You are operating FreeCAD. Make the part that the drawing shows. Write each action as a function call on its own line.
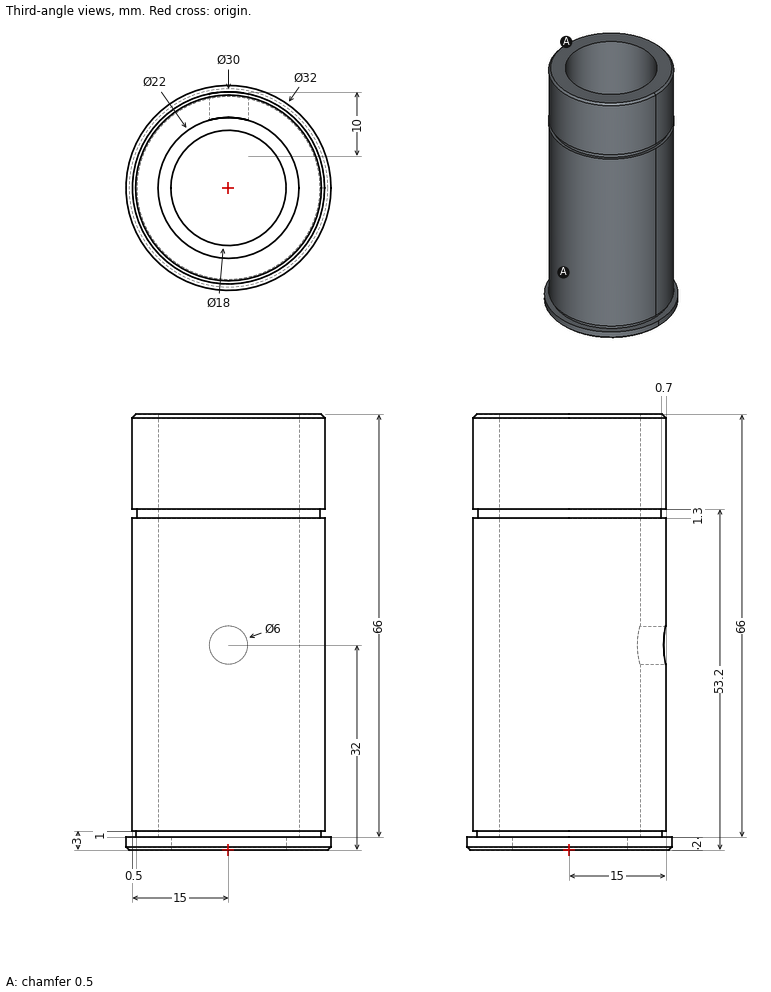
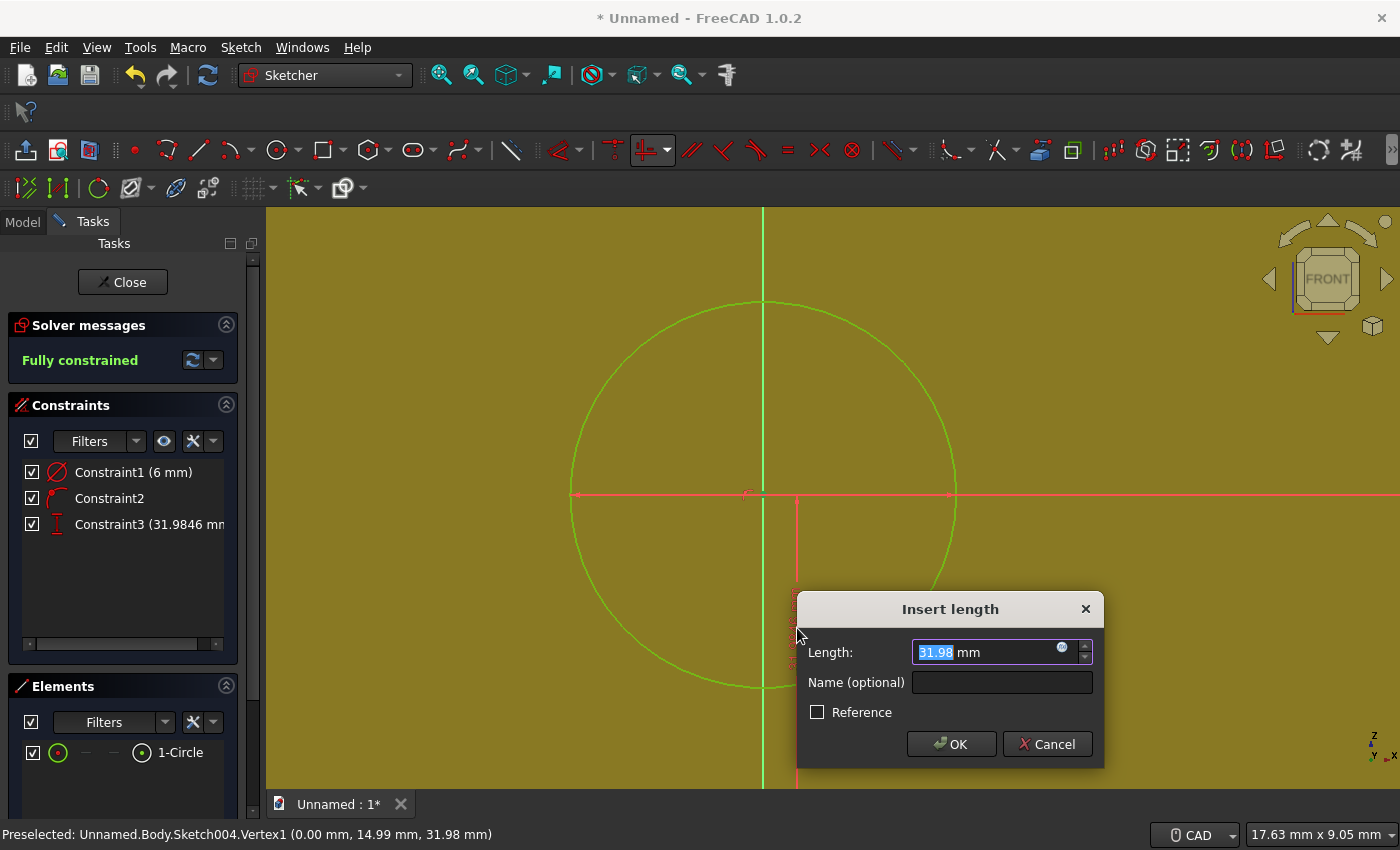
text(32)
key(Return)
key(Escape)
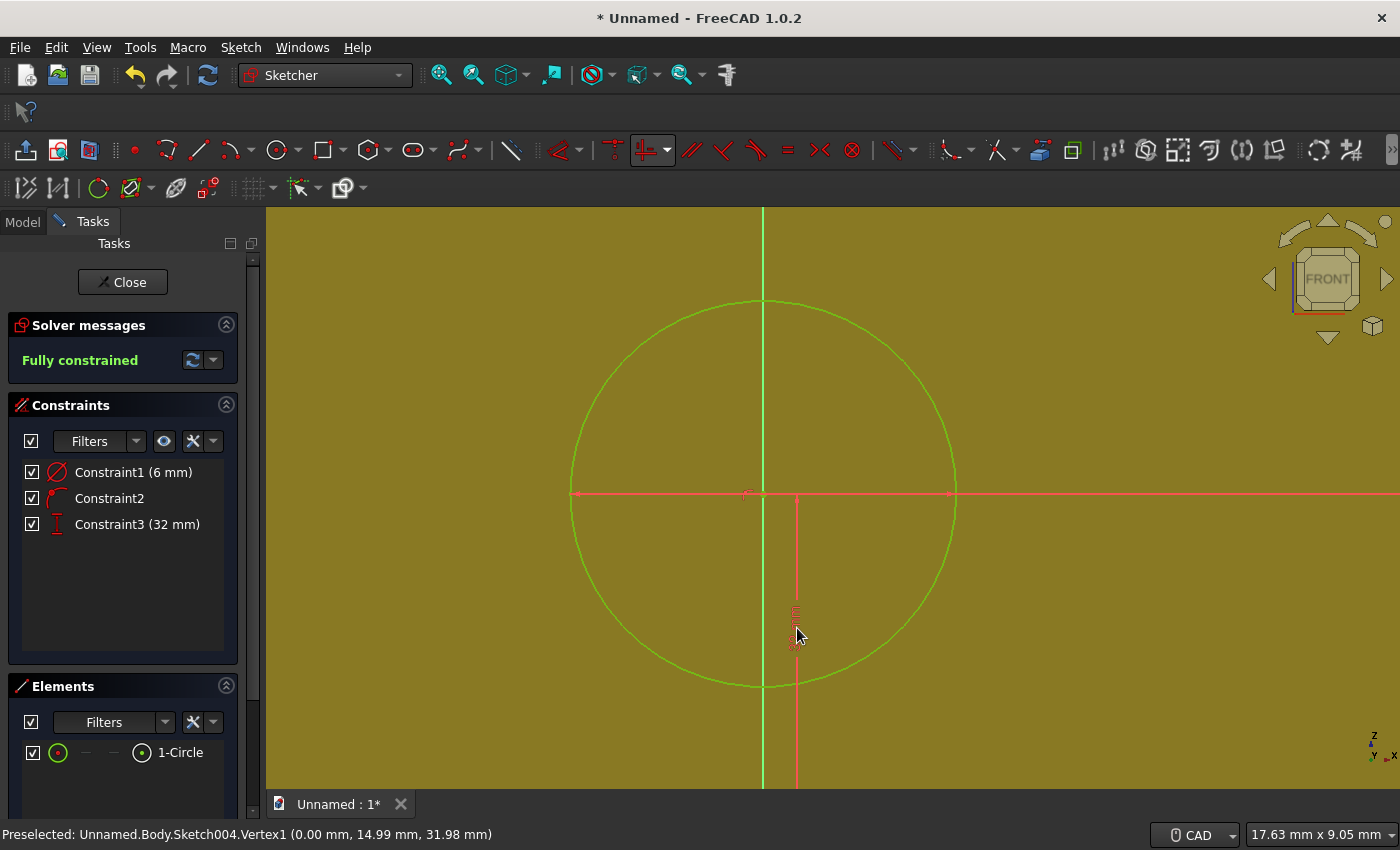
click(123, 282)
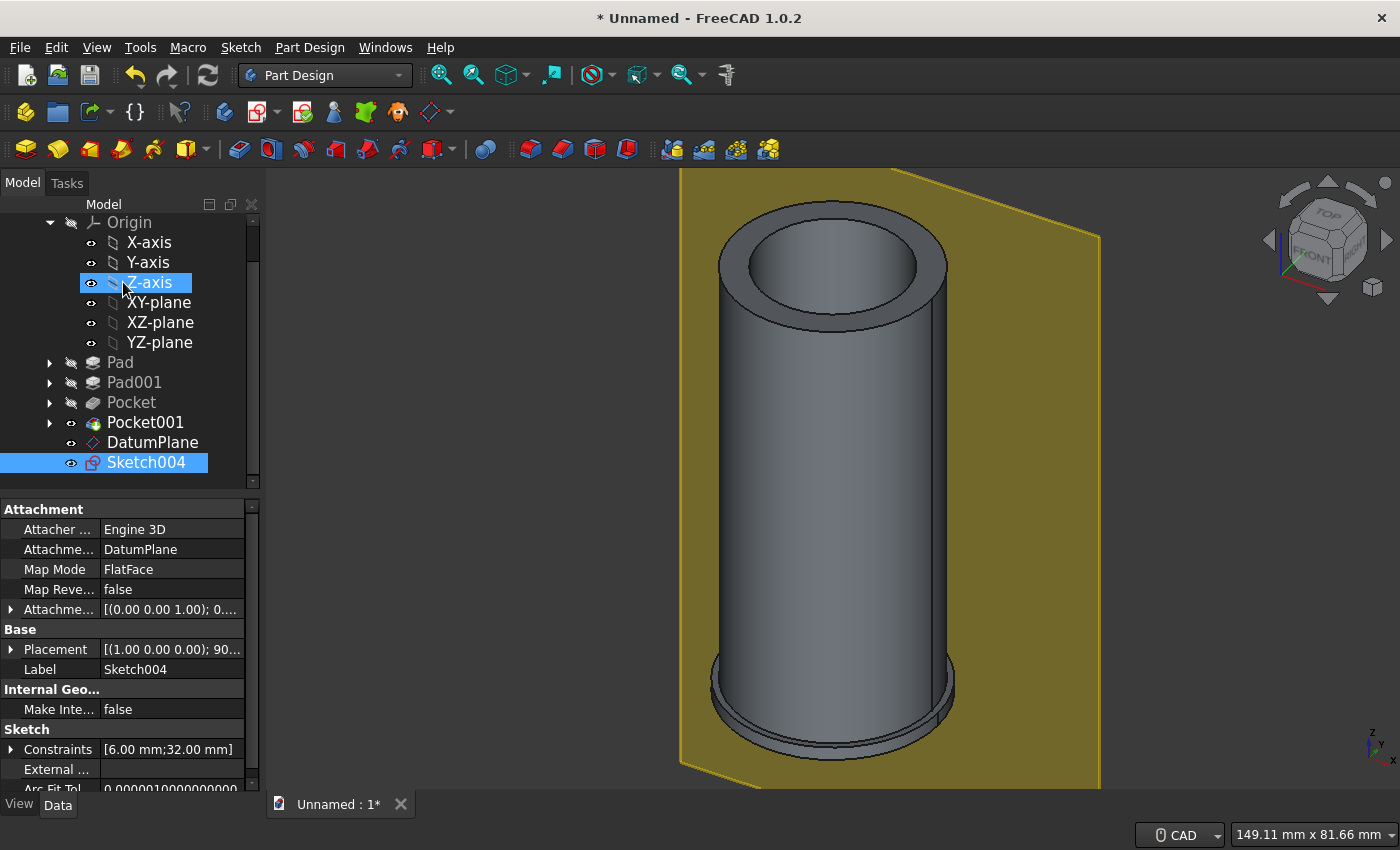
click(240, 150)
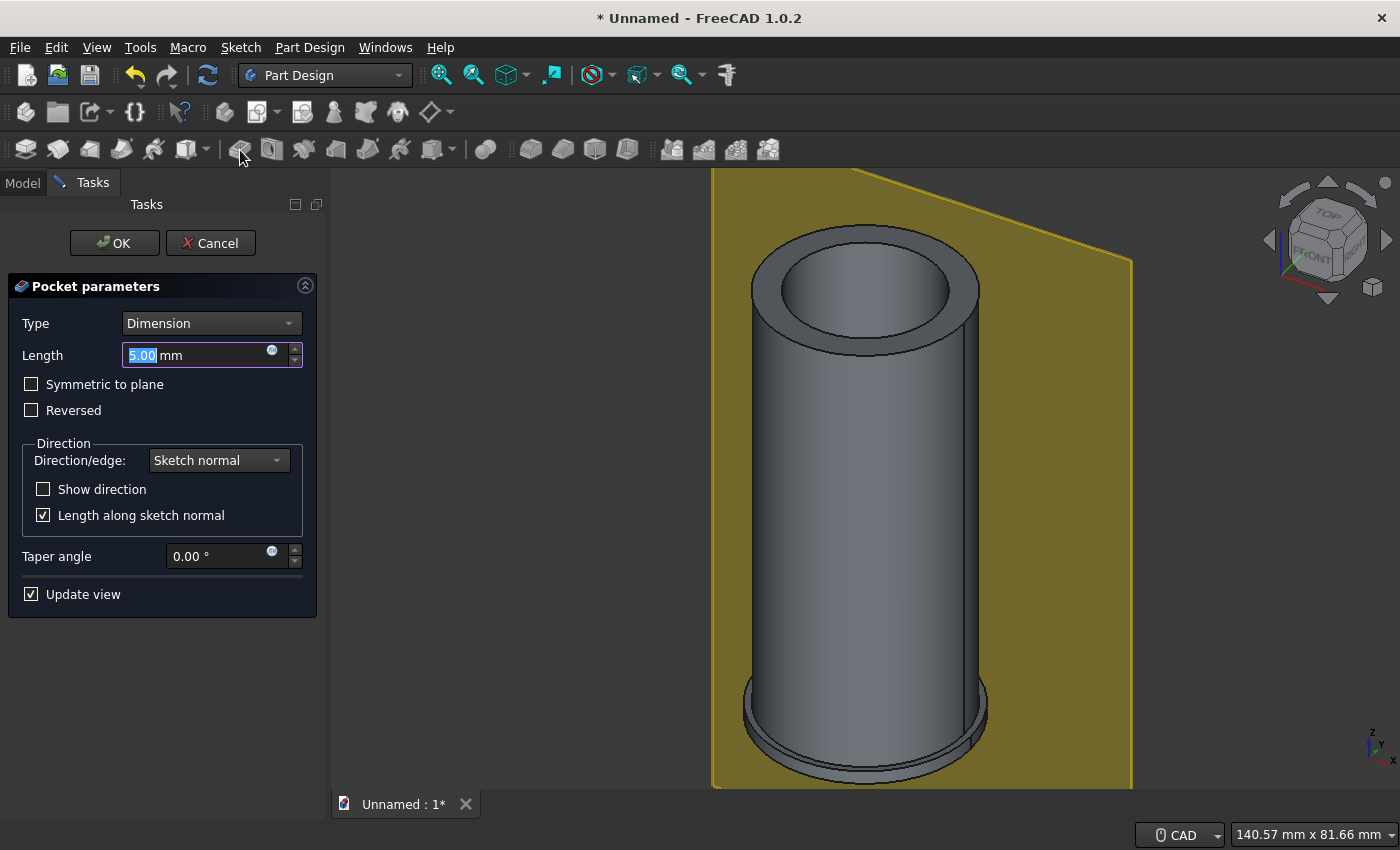
text(10)
key(Tab)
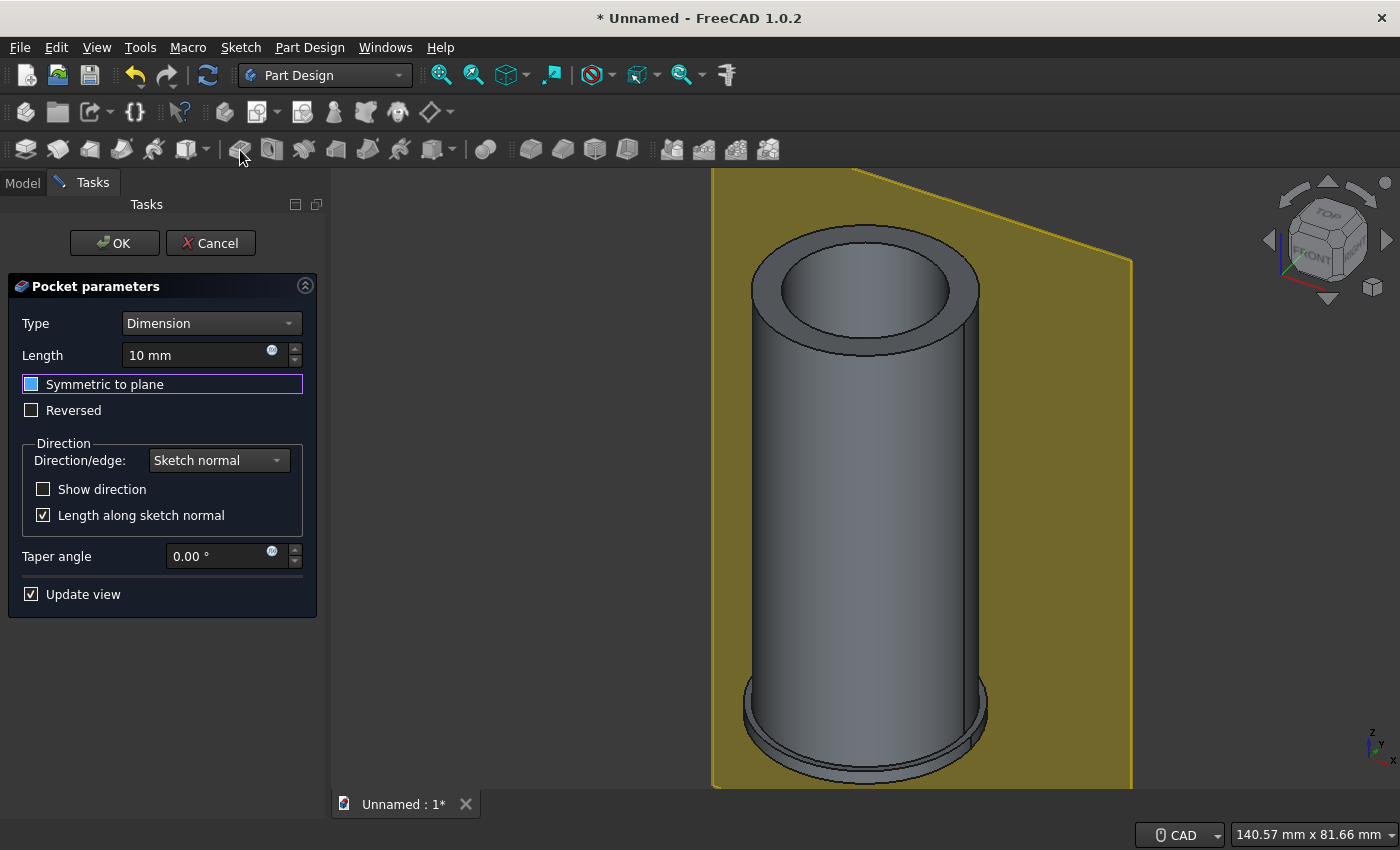
click(30, 410)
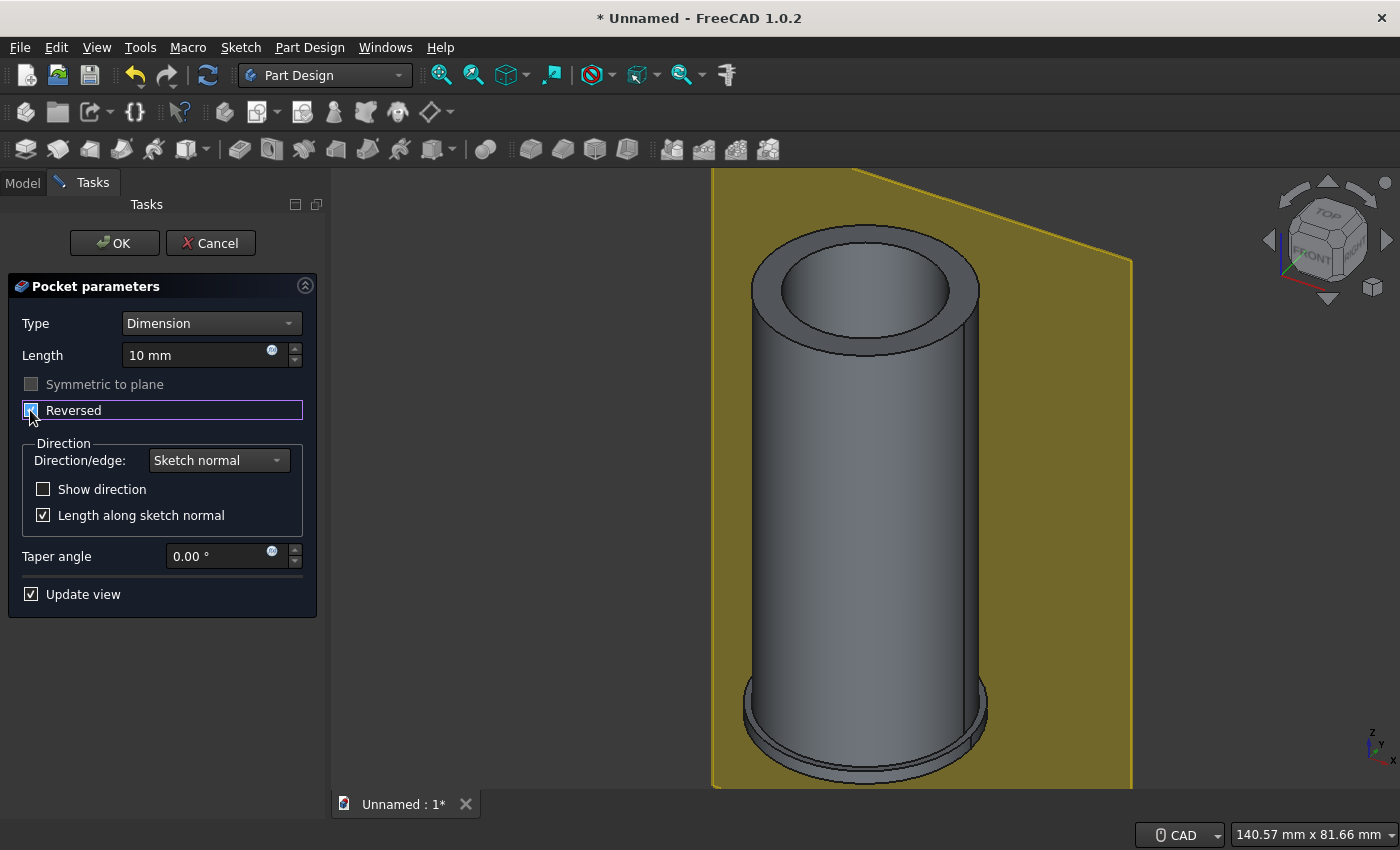
click(115, 243)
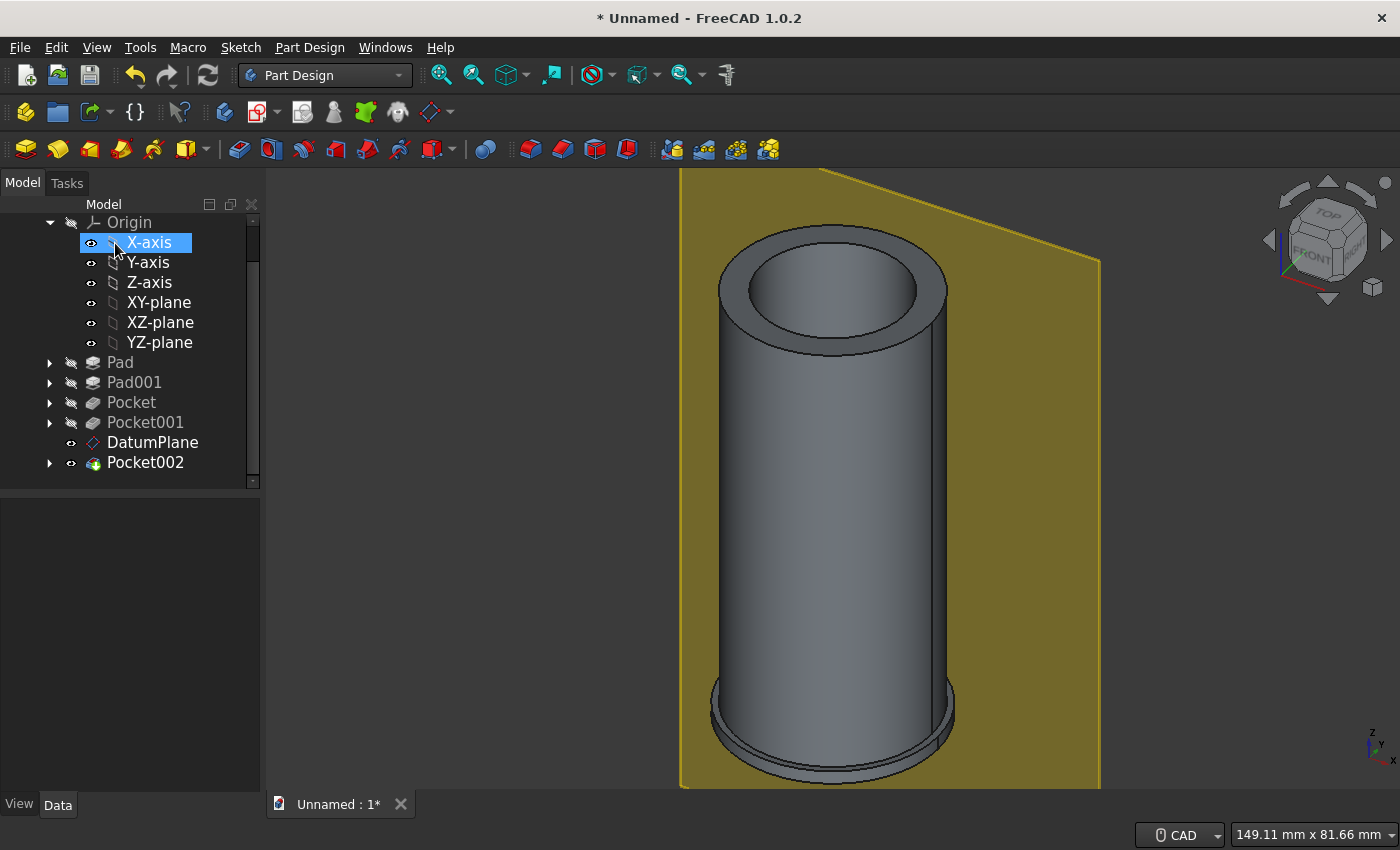
click(116, 443)
key(space)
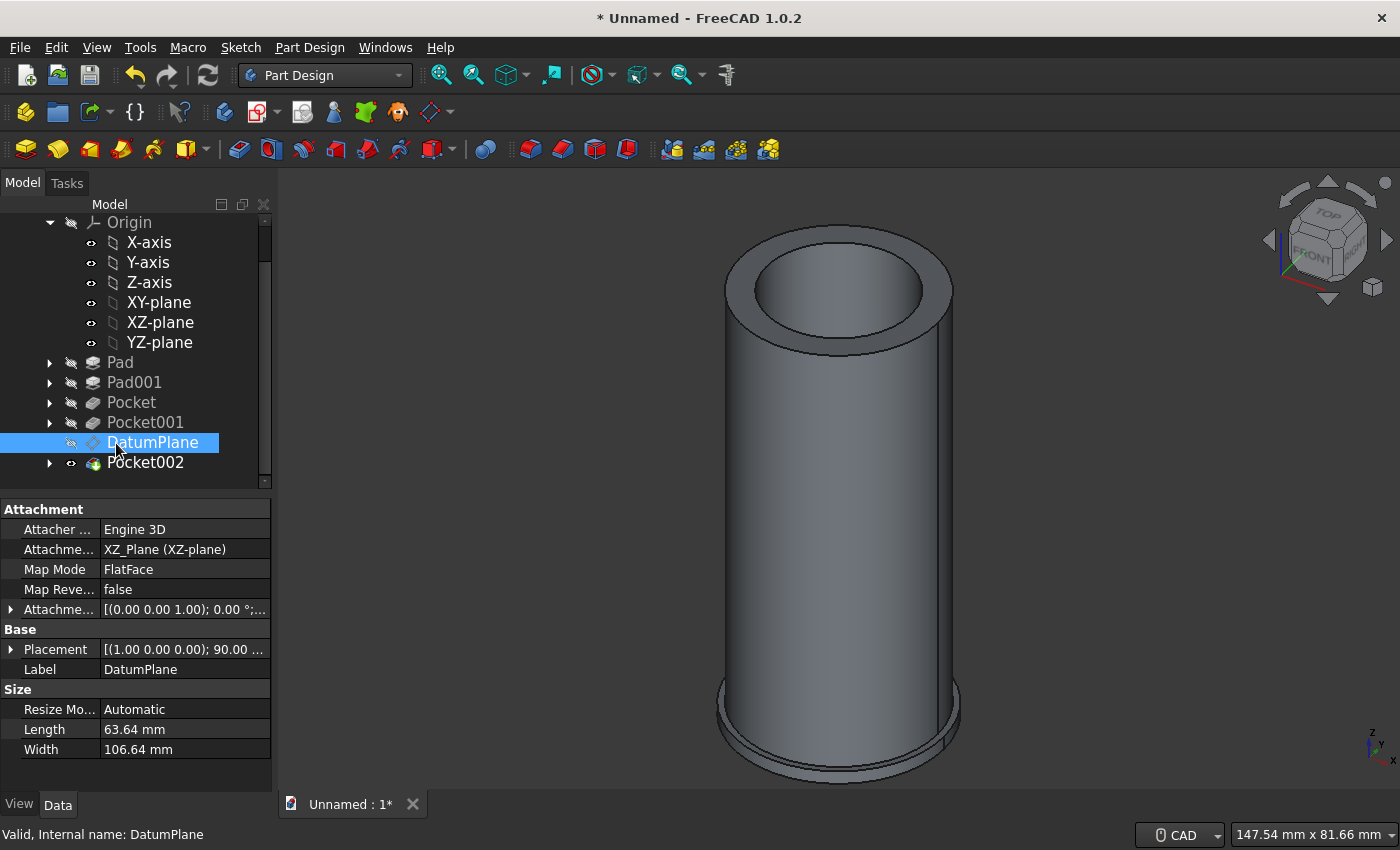
key(v)
key(f)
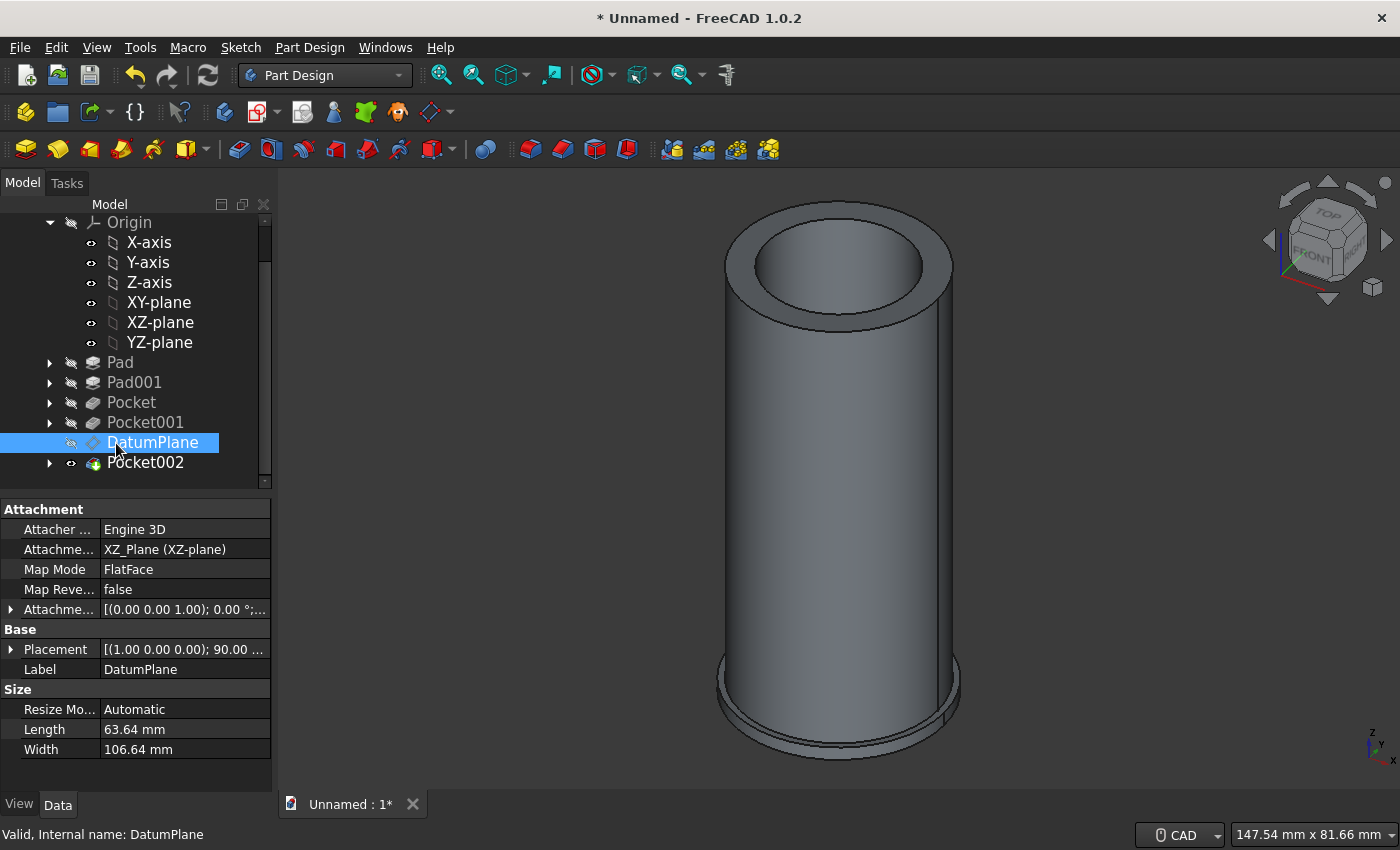
click(318, 749)